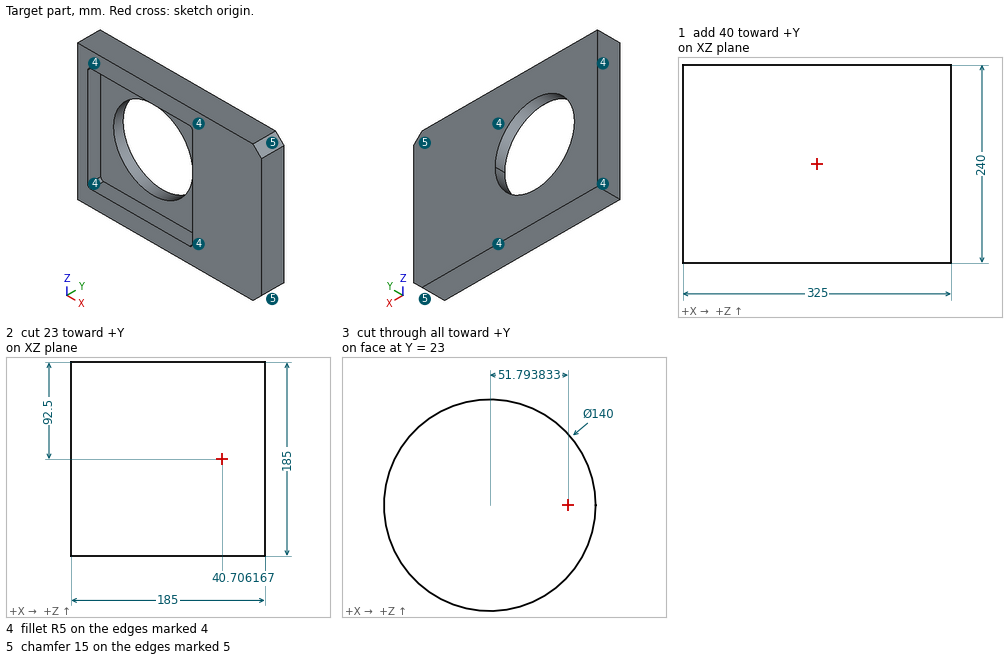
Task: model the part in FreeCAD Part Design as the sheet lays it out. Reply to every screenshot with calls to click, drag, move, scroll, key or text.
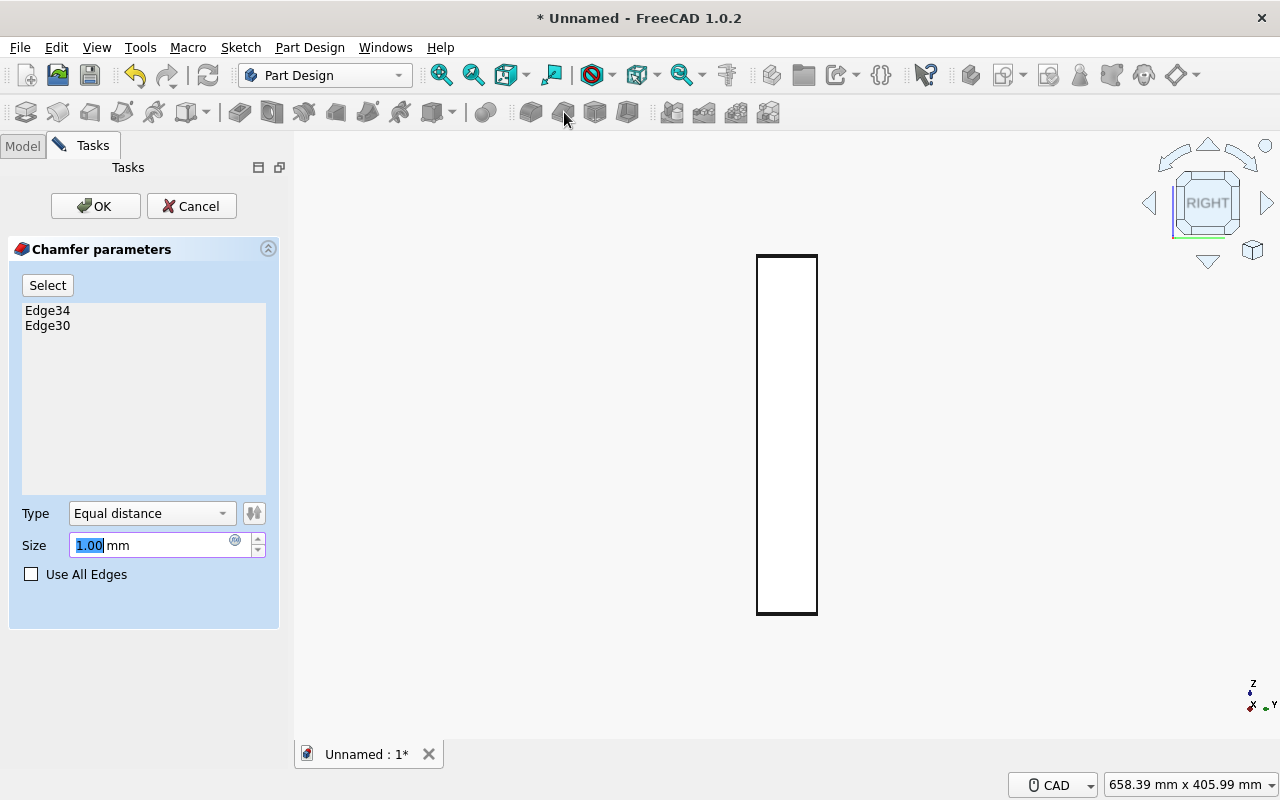
text(15)
key(Tab)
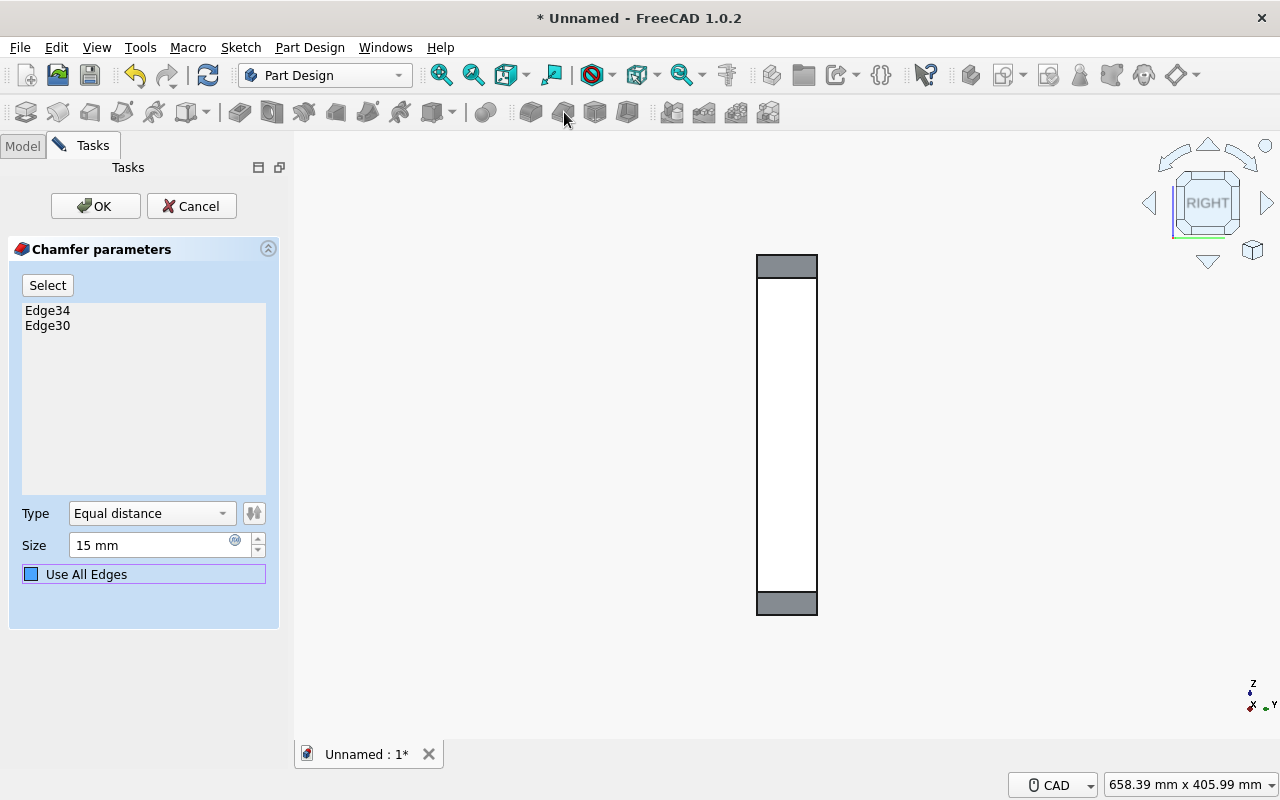
click(96, 206)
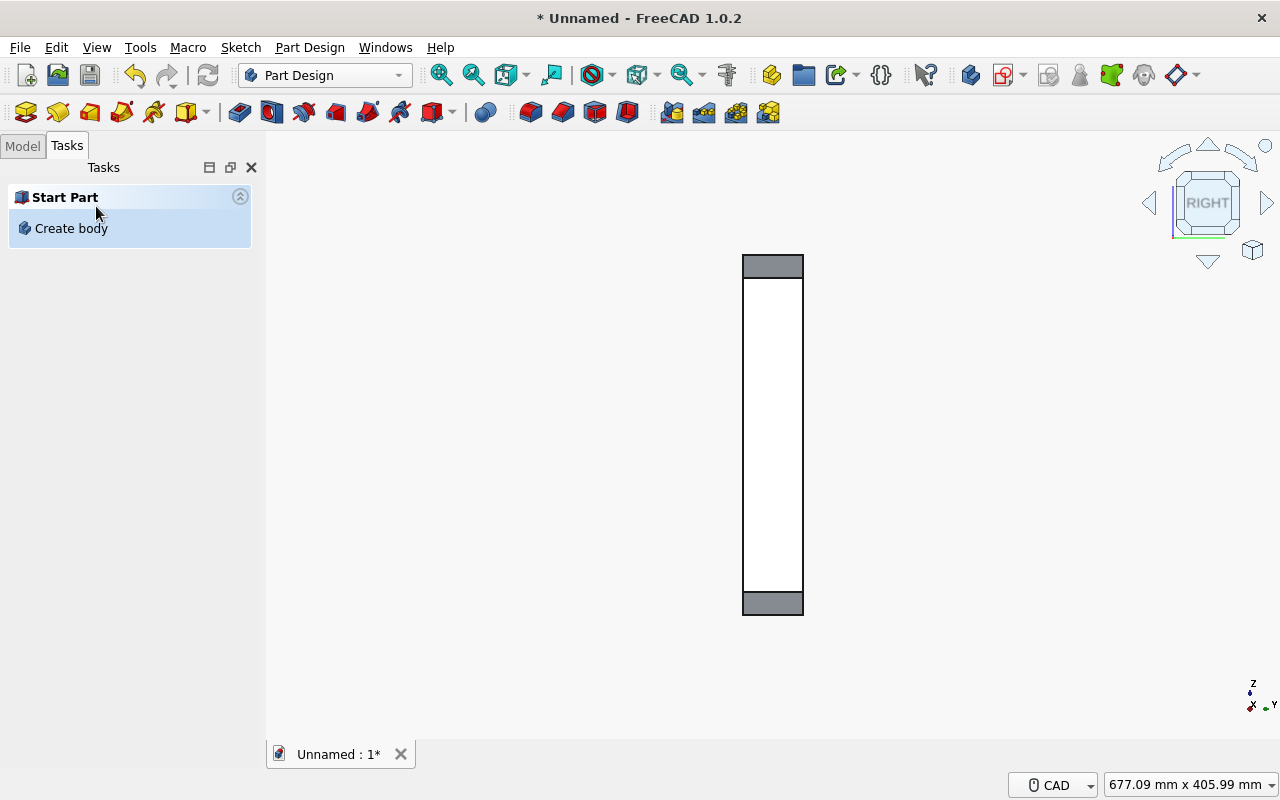
key(0)